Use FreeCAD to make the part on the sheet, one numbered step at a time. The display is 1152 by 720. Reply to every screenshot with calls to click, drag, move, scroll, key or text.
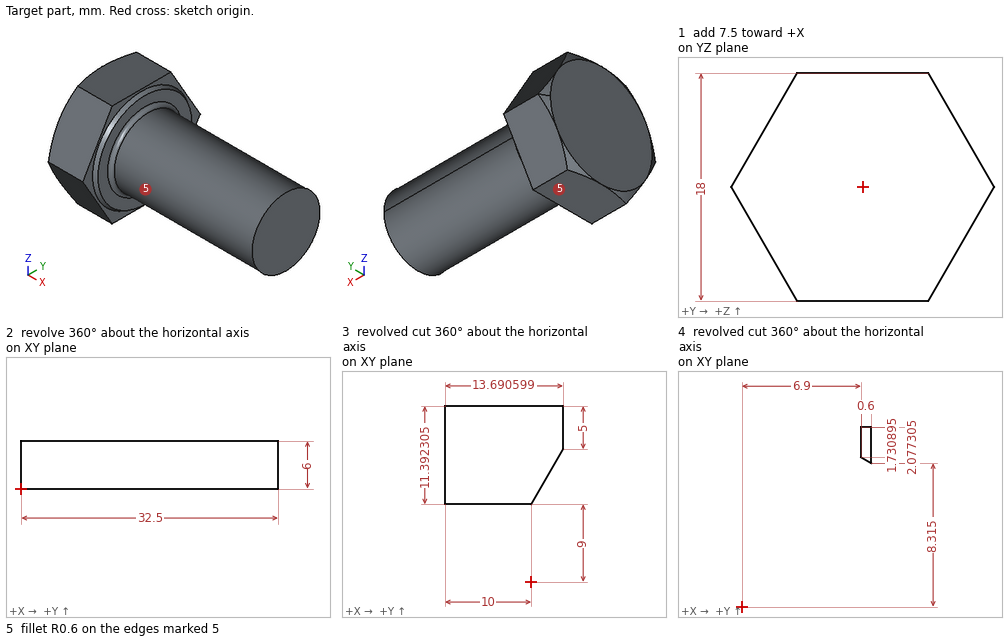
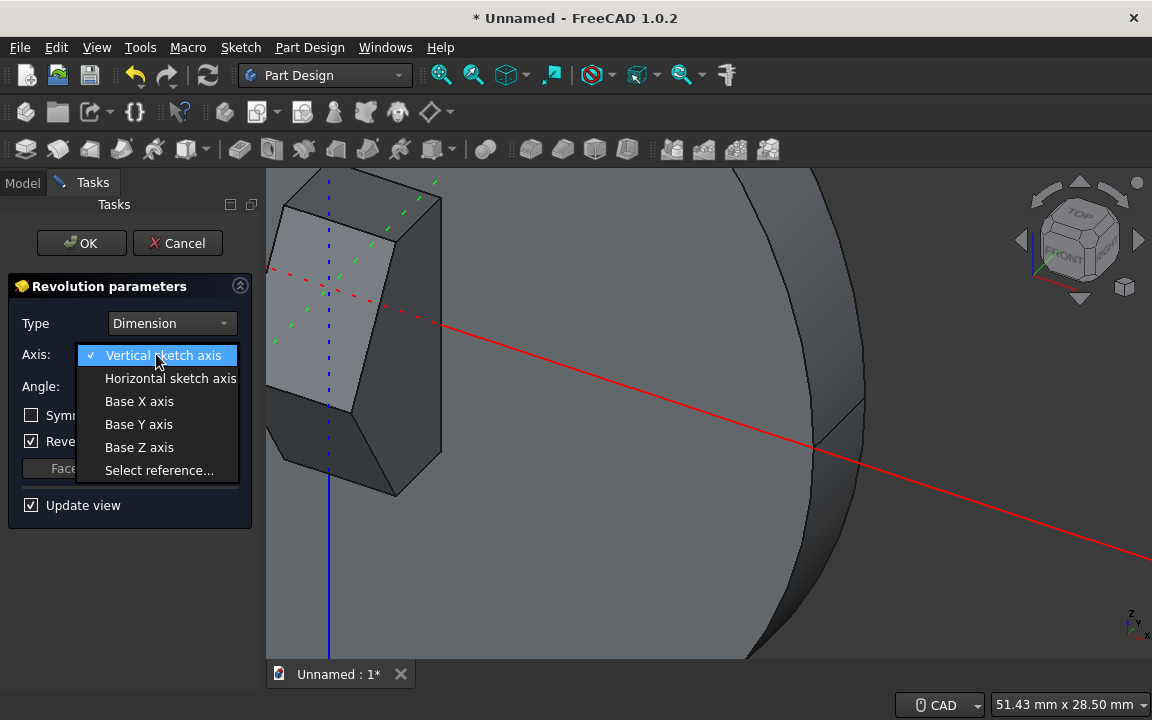
click(156, 378)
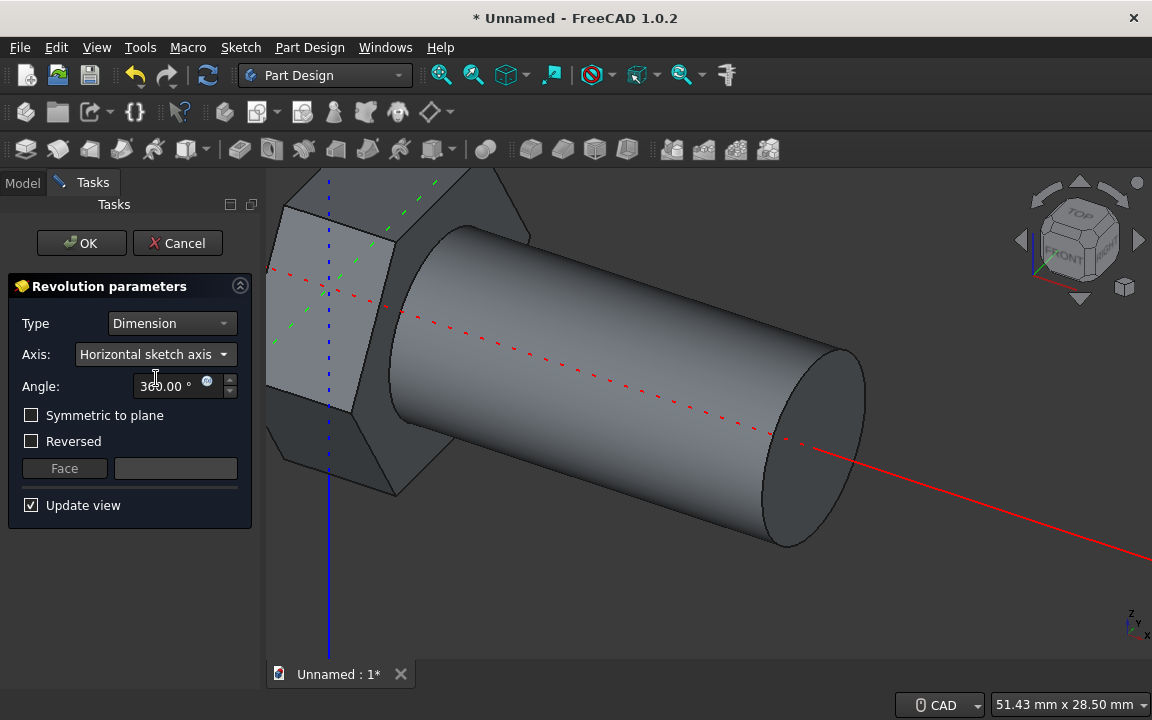
click(82, 243)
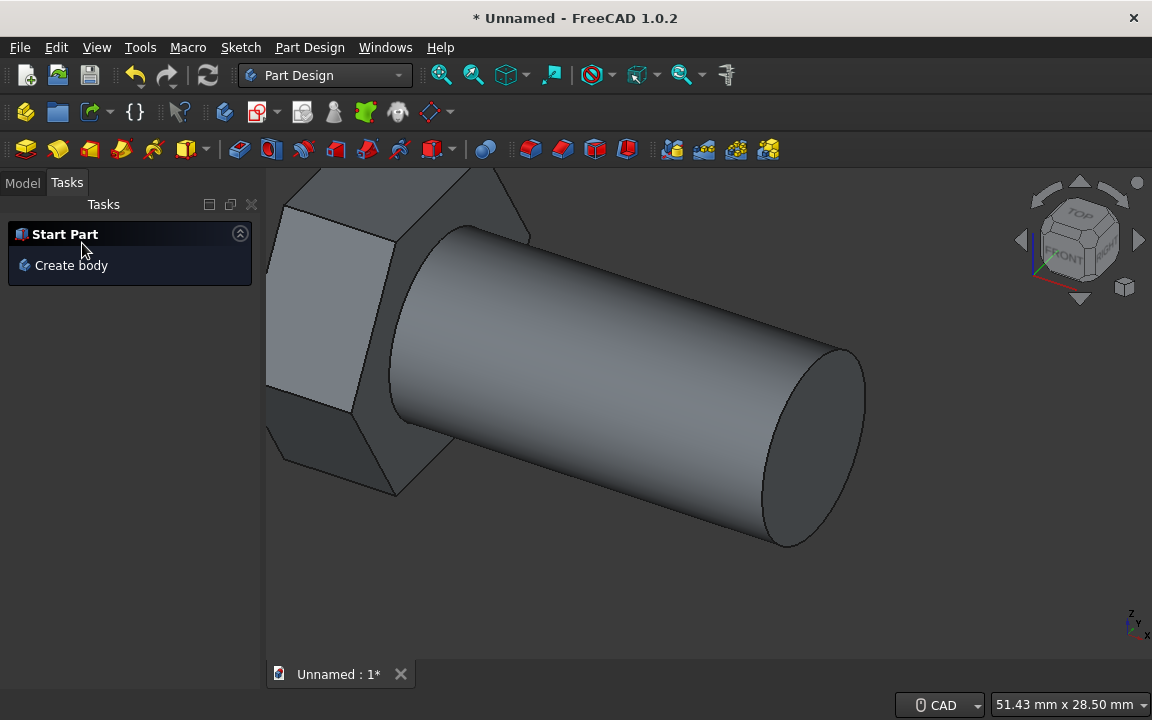
click(442, 76)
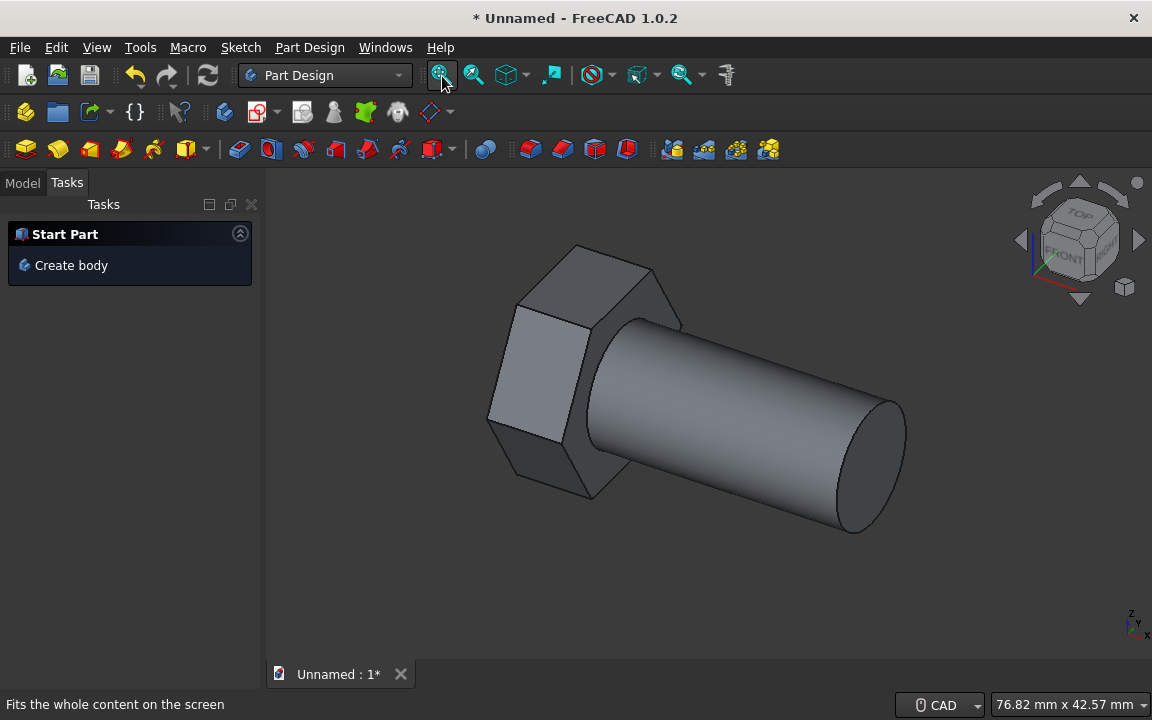
click(258, 112)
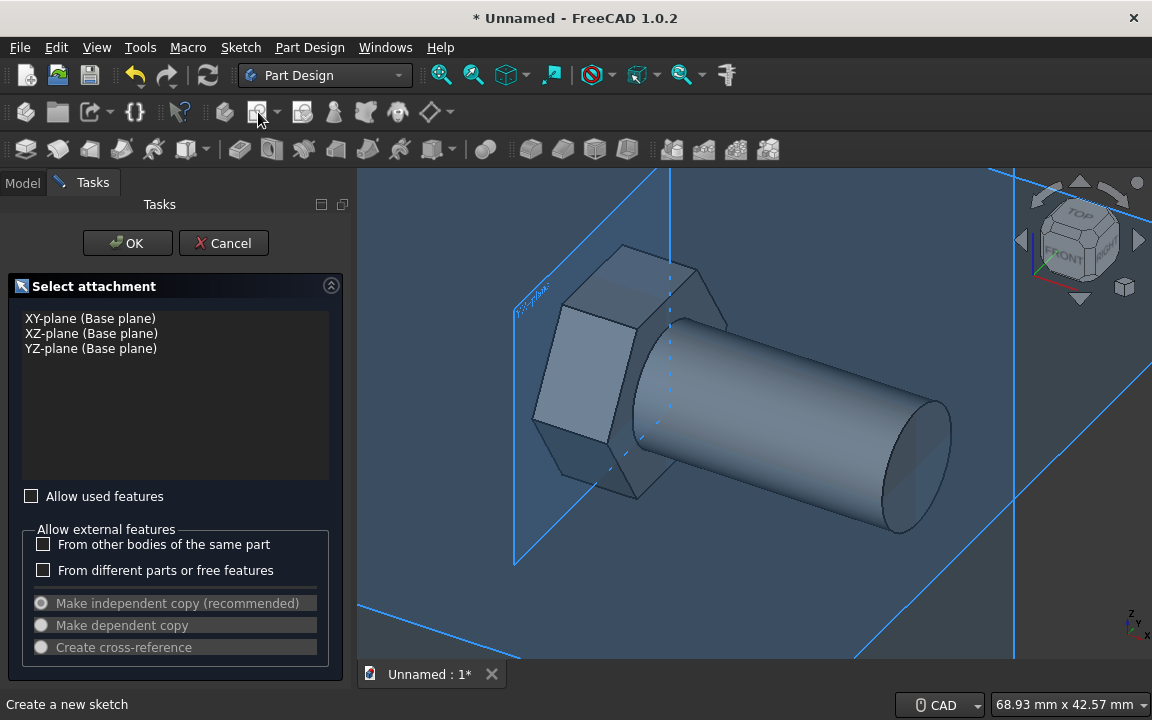
click(82, 318)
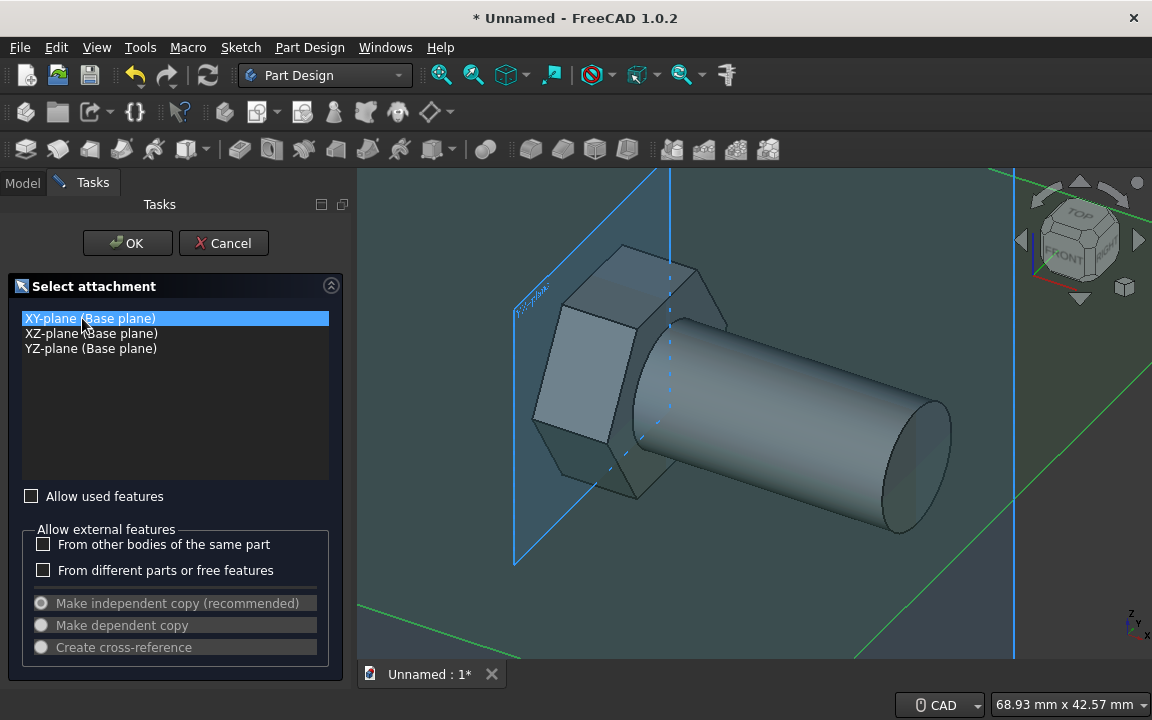
click(128, 243)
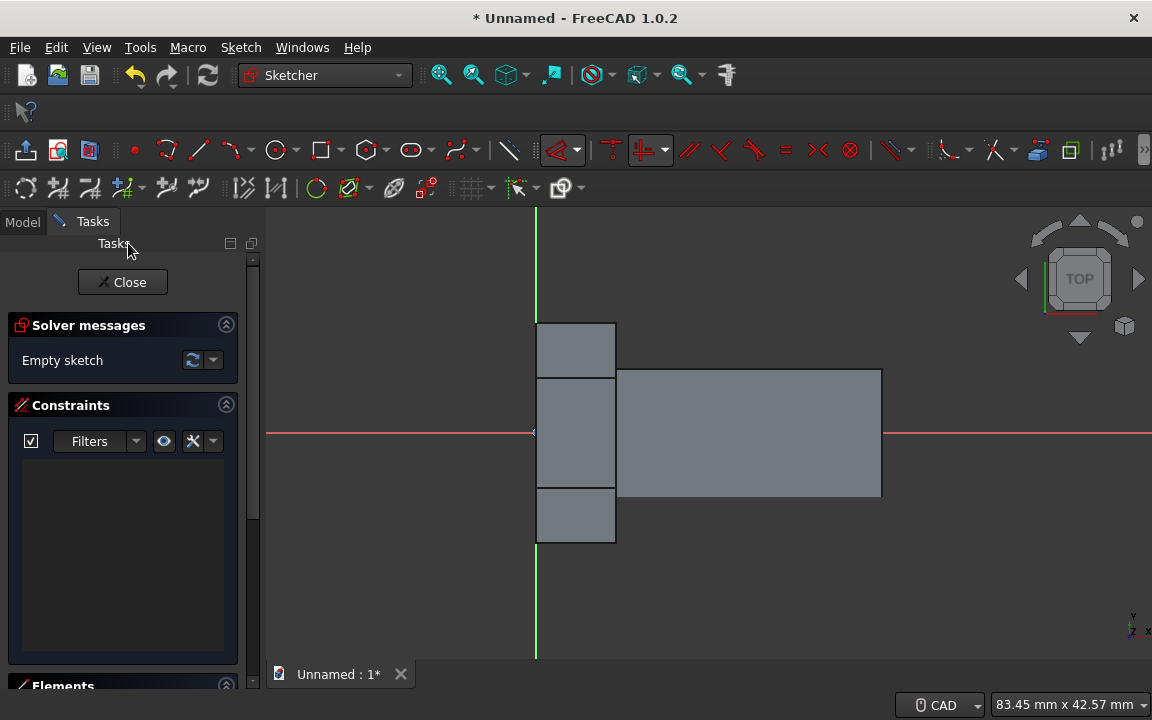
click(90, 150)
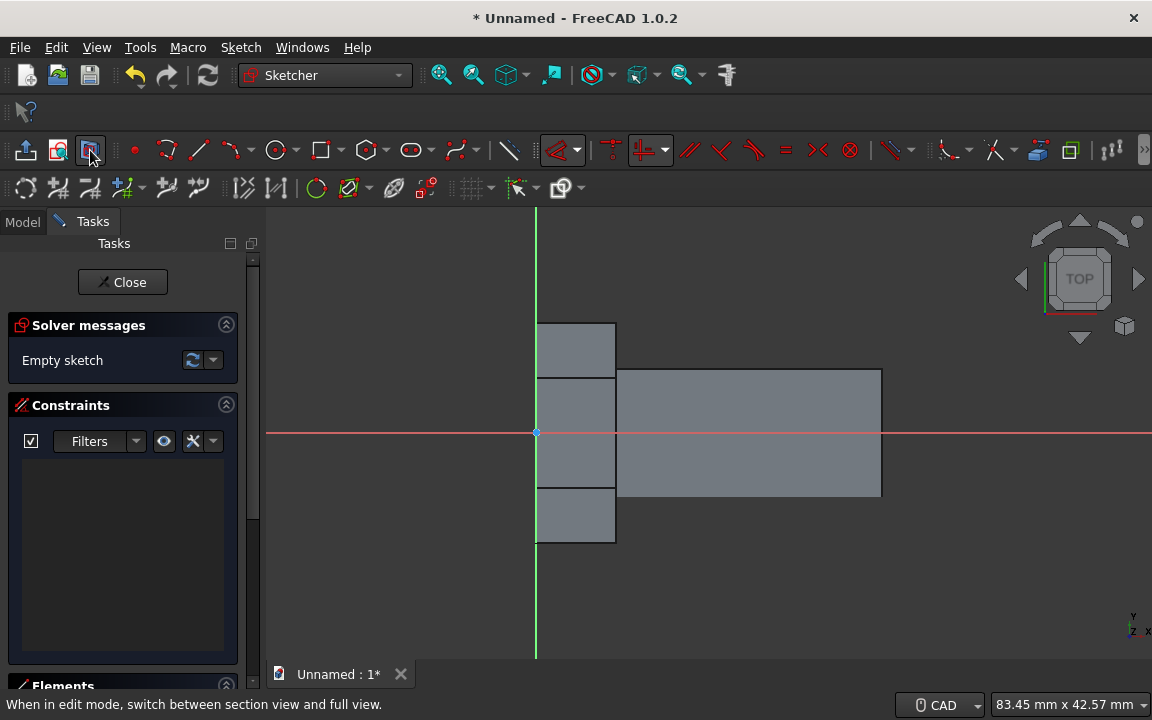
scroll(987, 631, down, 1)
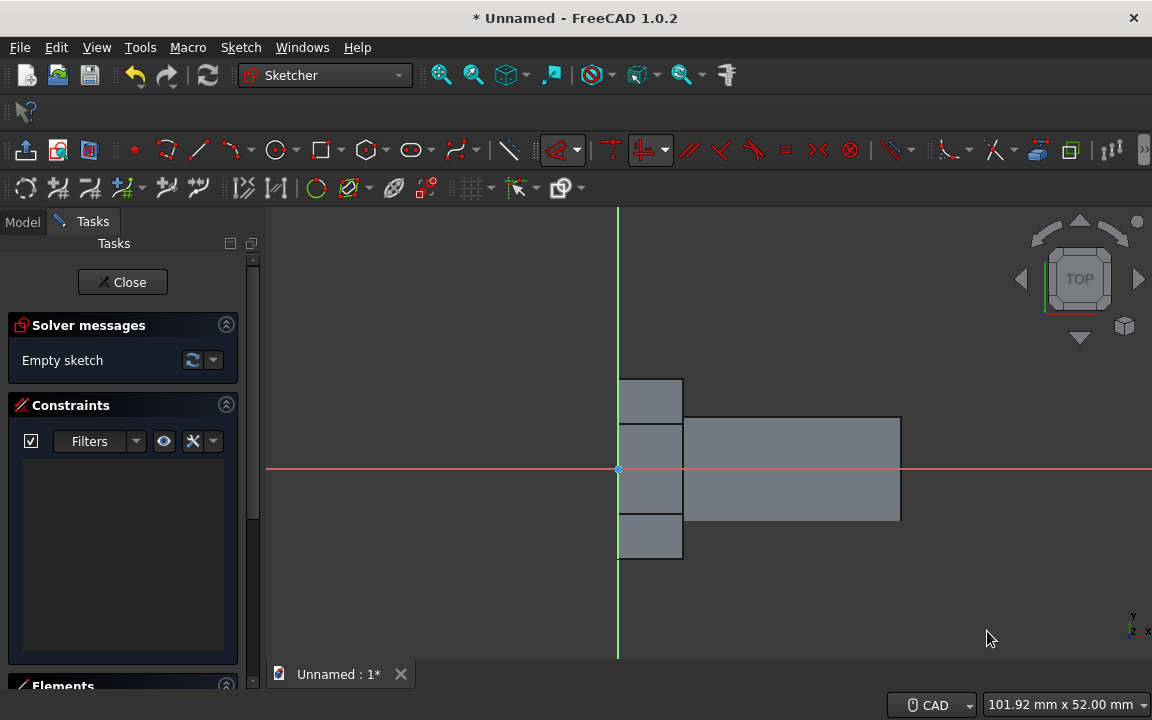
scroll(490, 274, up, 2)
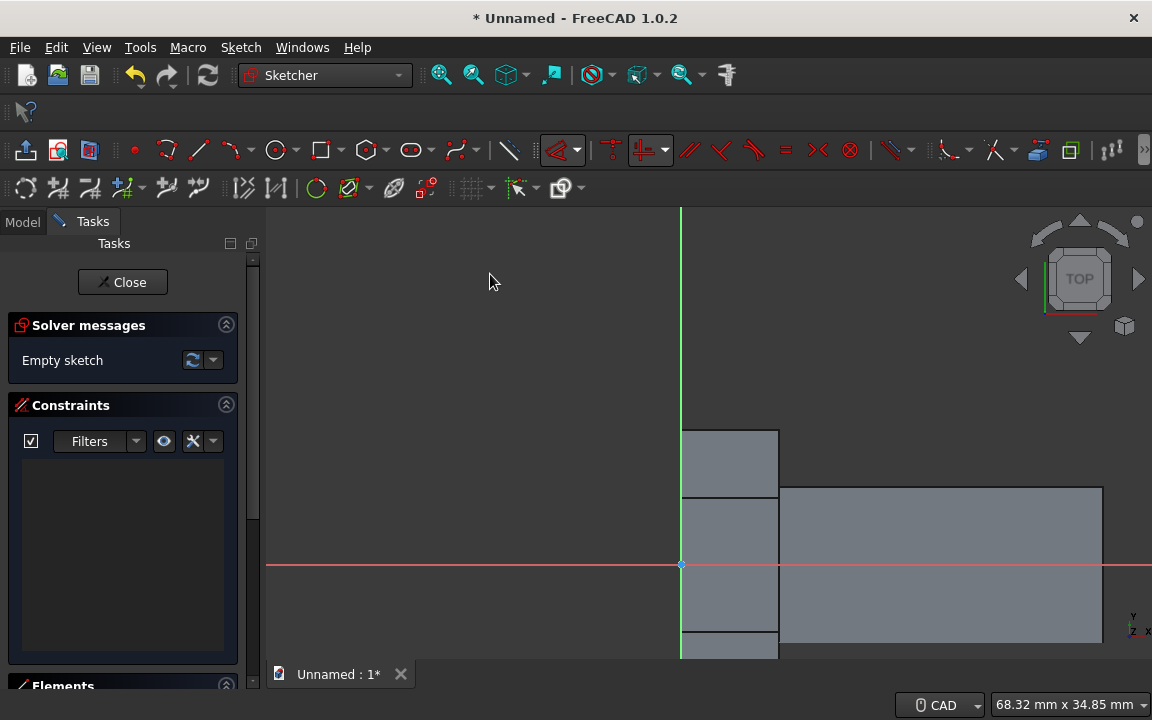
click(168, 150)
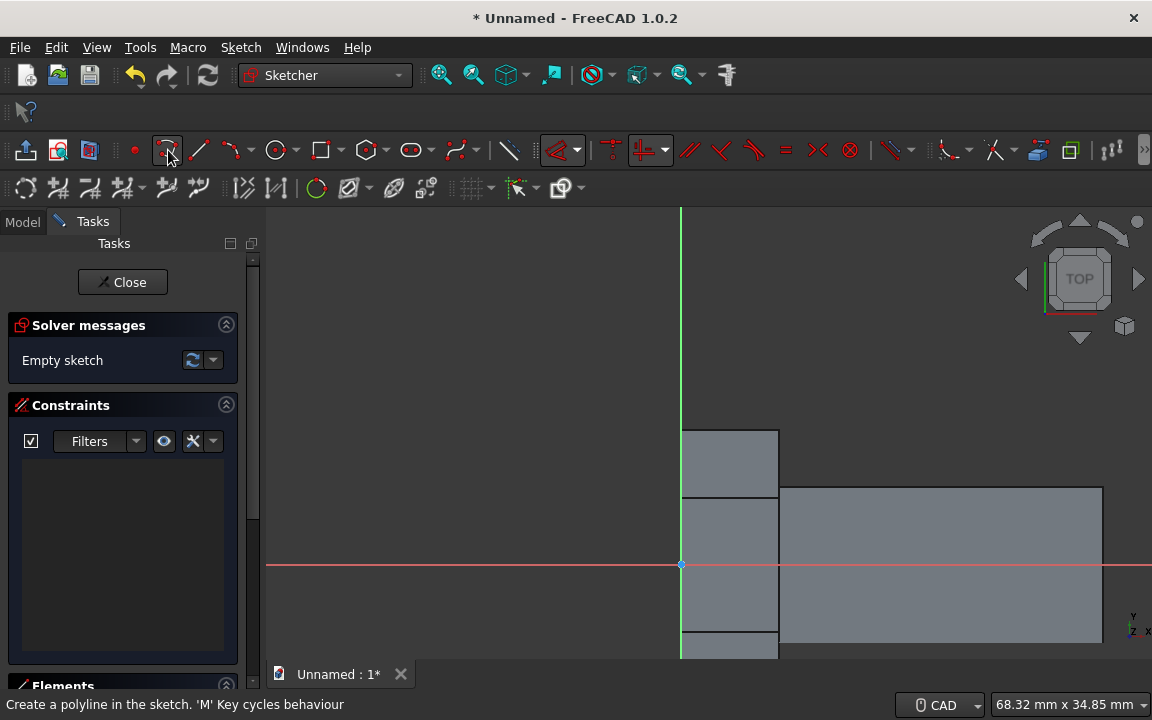
click(681, 448)
click(729, 365)
click(729, 300)
click(552, 300)
click(552, 448)
click(681, 449)
key(Escape)
key(Escape)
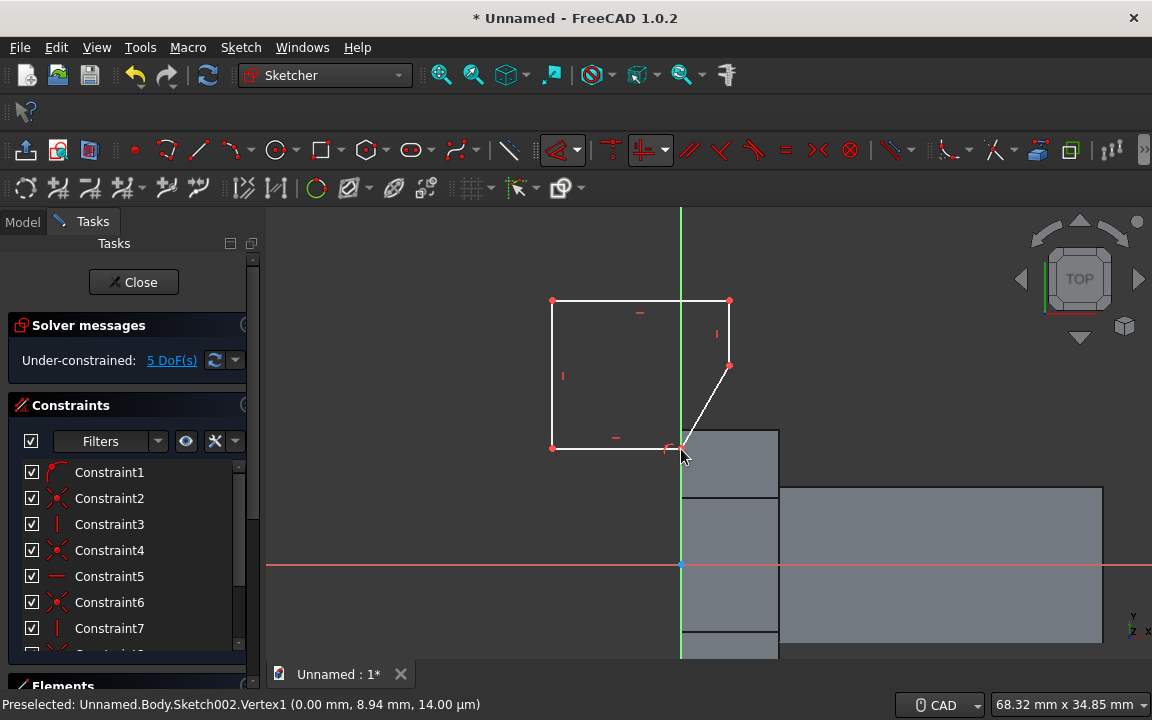
click(729, 347)